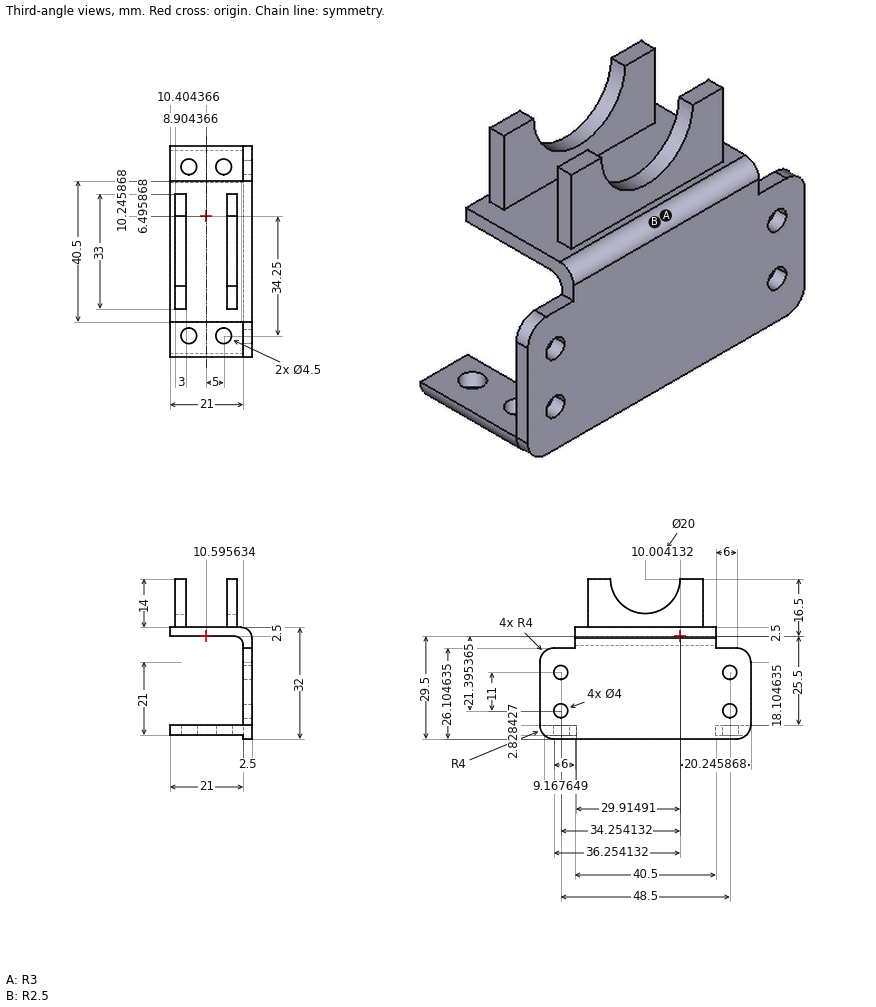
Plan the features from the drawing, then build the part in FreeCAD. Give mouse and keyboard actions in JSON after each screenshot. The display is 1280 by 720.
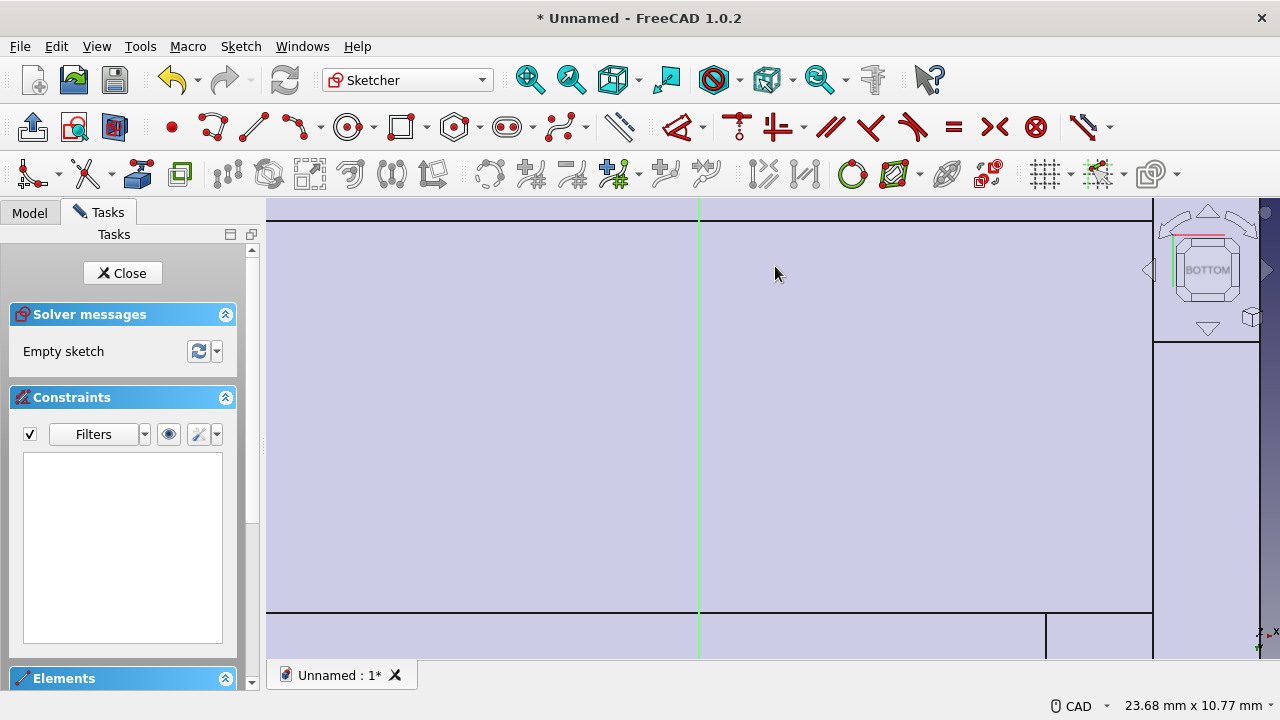
{"action": "left_click", "coordinate": [348, 128]}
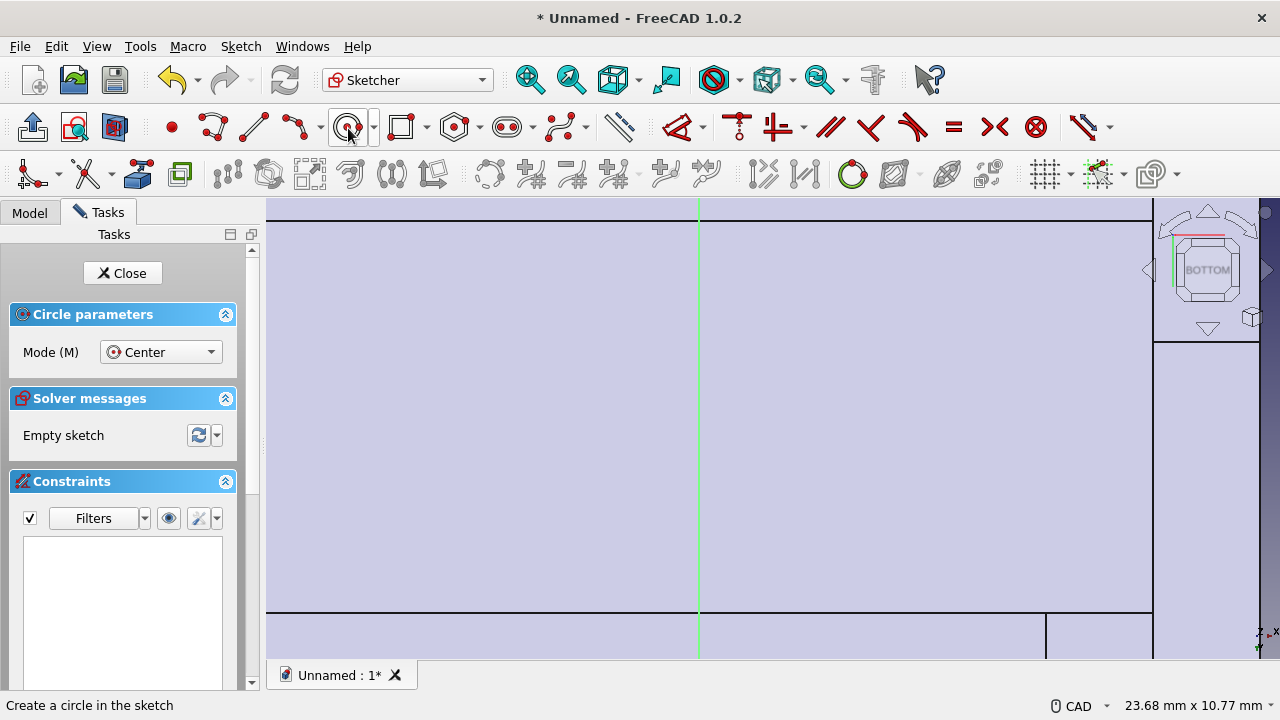
{"action": "left_click", "coordinate": [913, 428]}
{"action": "left_click", "coordinate": [982, 359]}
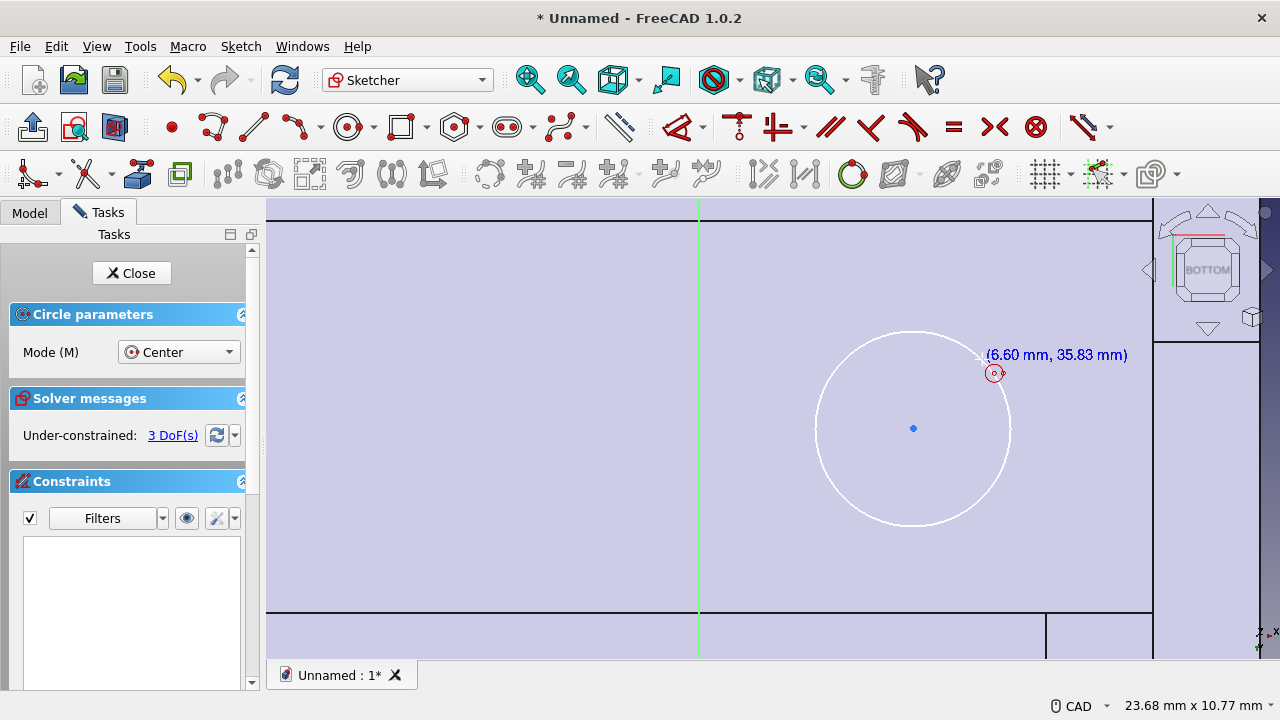
{"action": "left_click", "coordinate": [485, 428]}
{"action": "left_click", "coordinate": [553, 359]}
{"action": "key", "text": "Escape"}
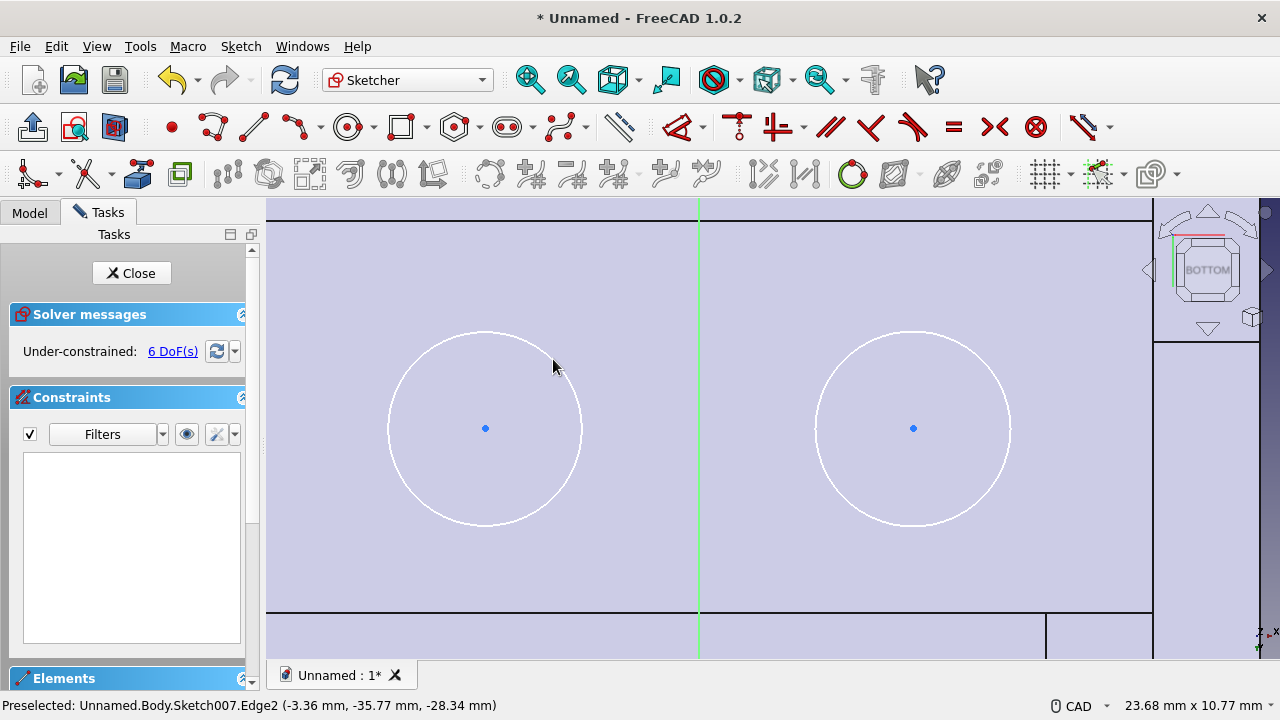
{"action": "left_click", "coordinate": [982, 360]}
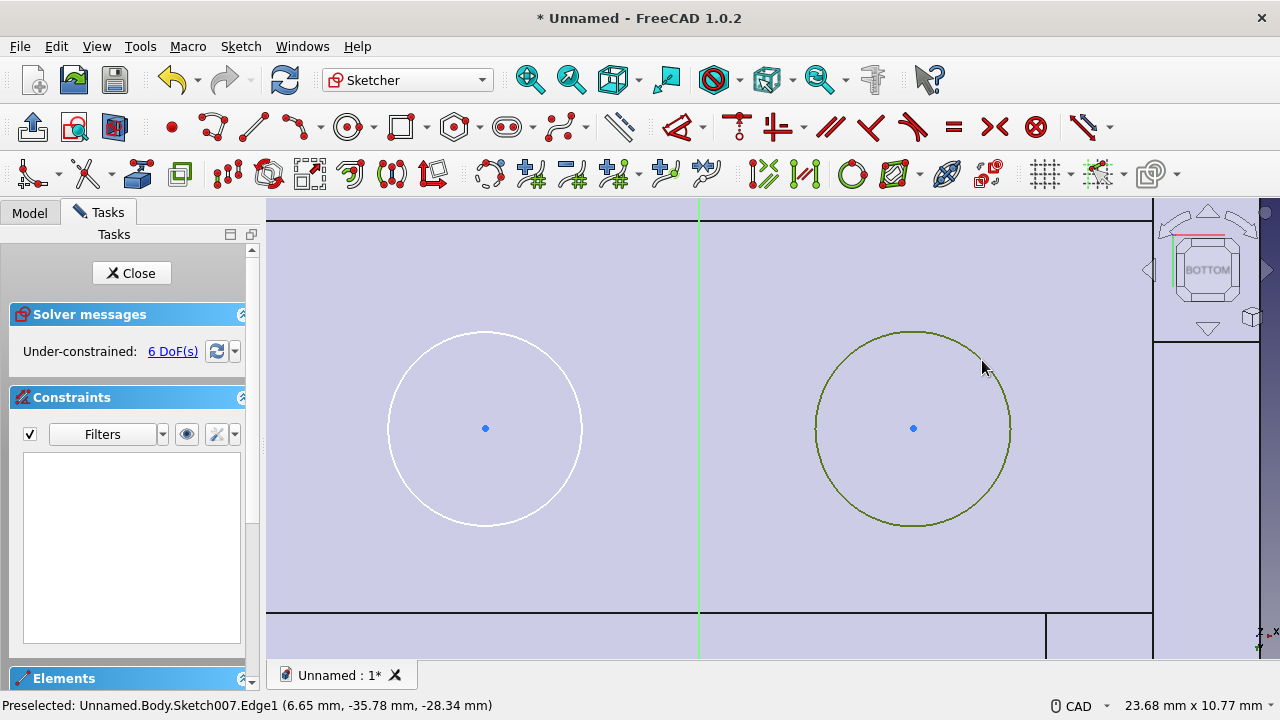
{"action": "left_click", "coordinate": [553, 360]}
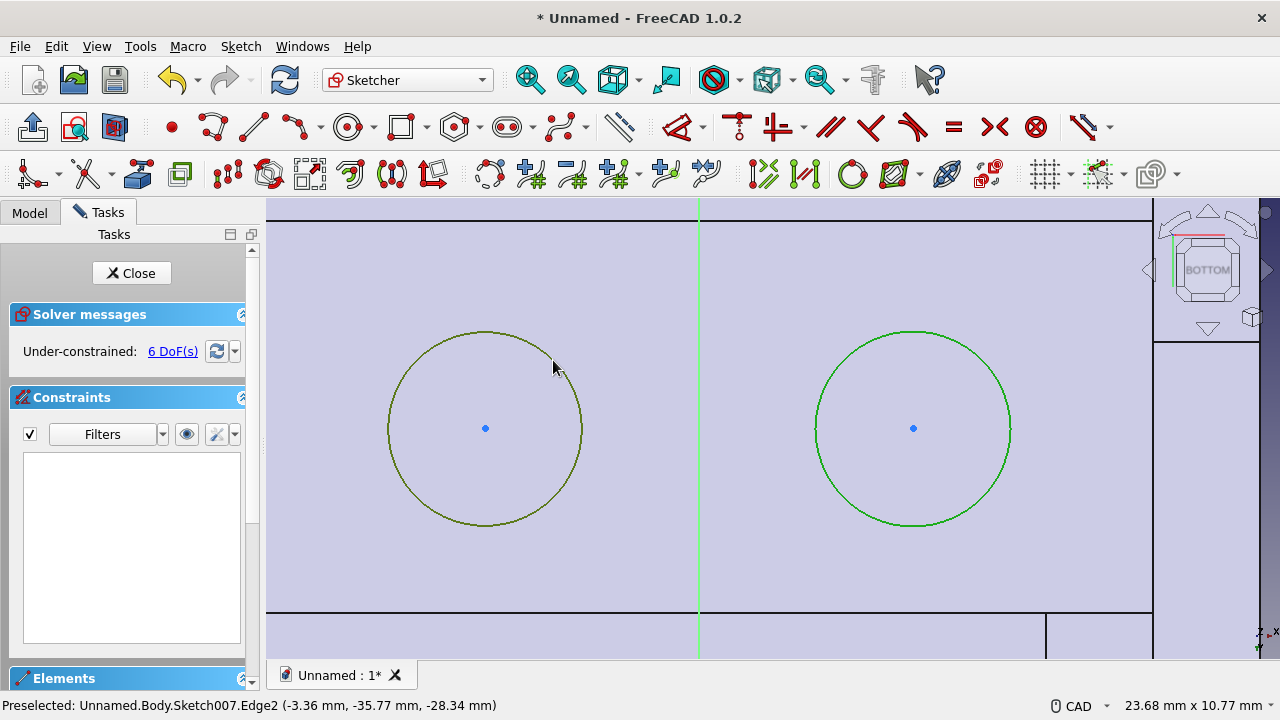
{"action": "left_click", "coordinate": [954, 128]}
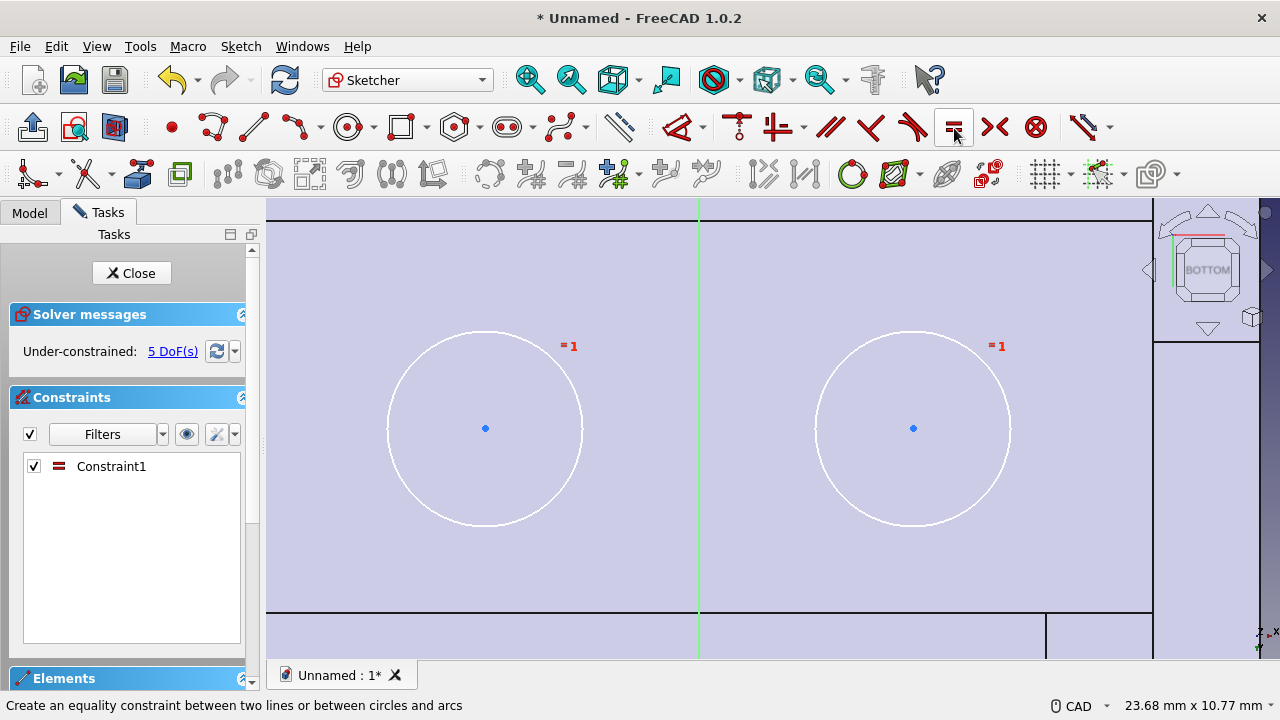
{"action": "left_click", "coordinate": [913, 429]}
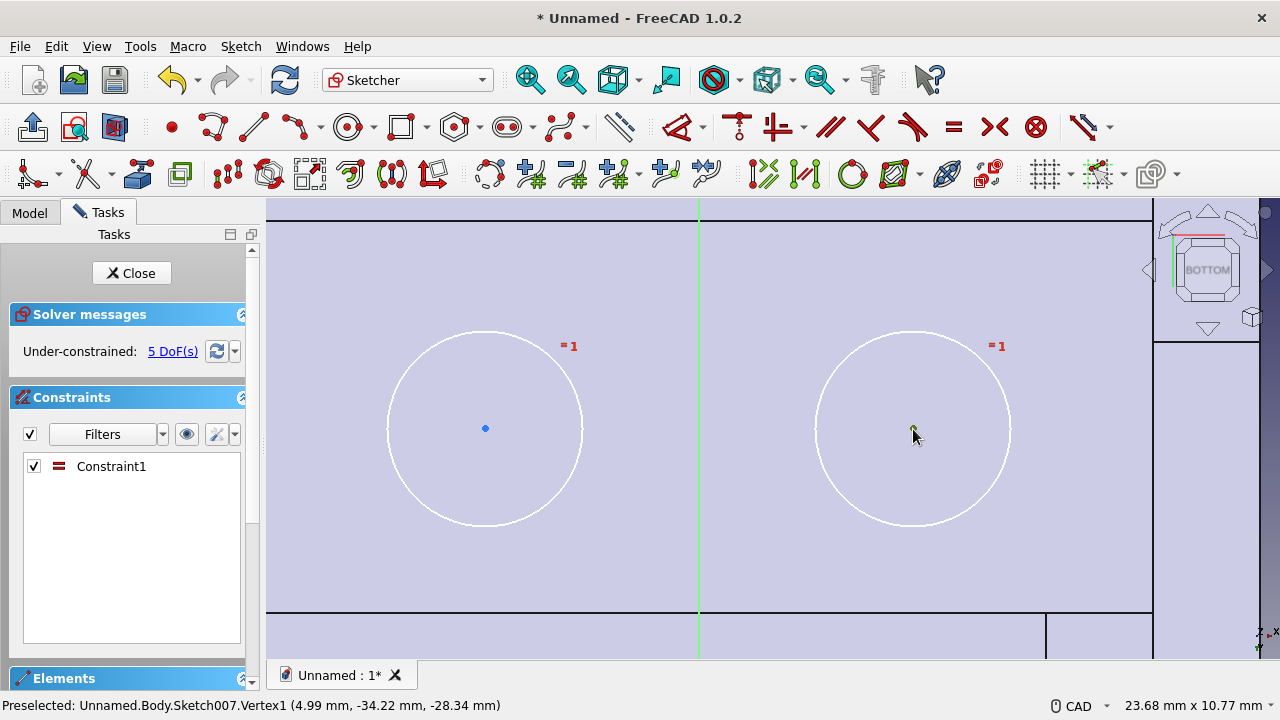
{"action": "left_click", "coordinate": [485, 429]}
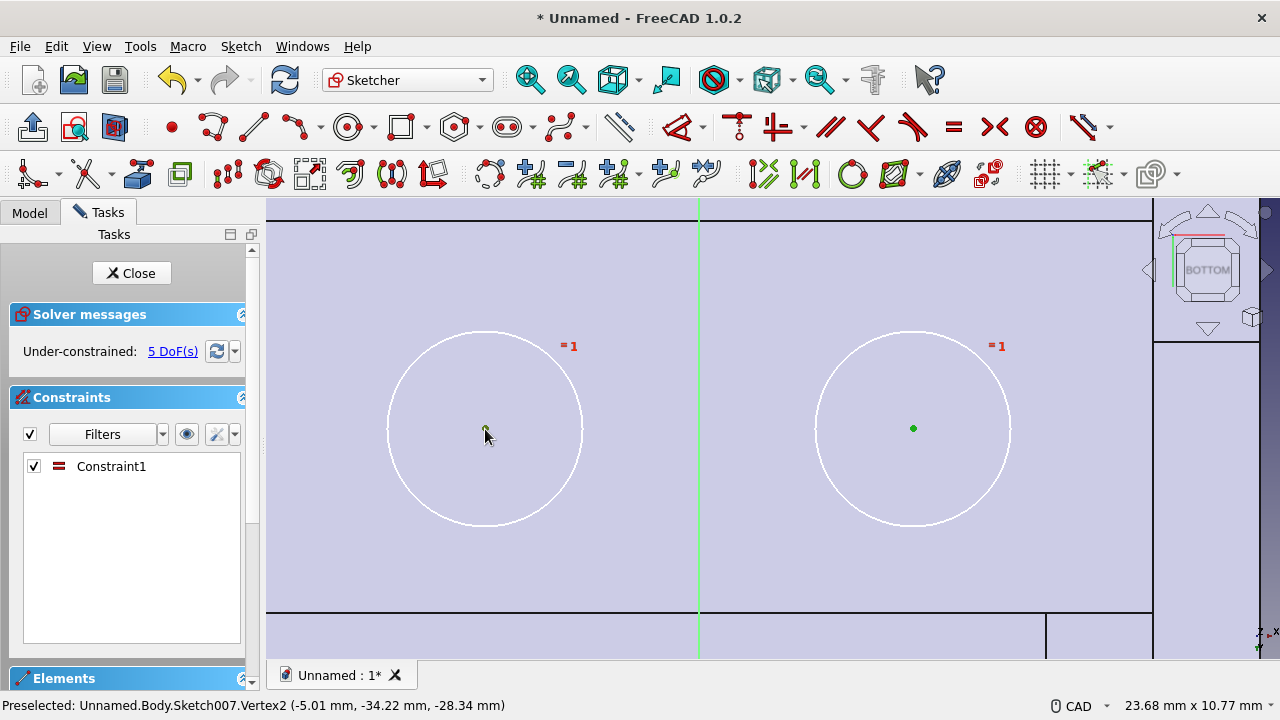
{"action": "left_click", "coordinate": [699, 602]}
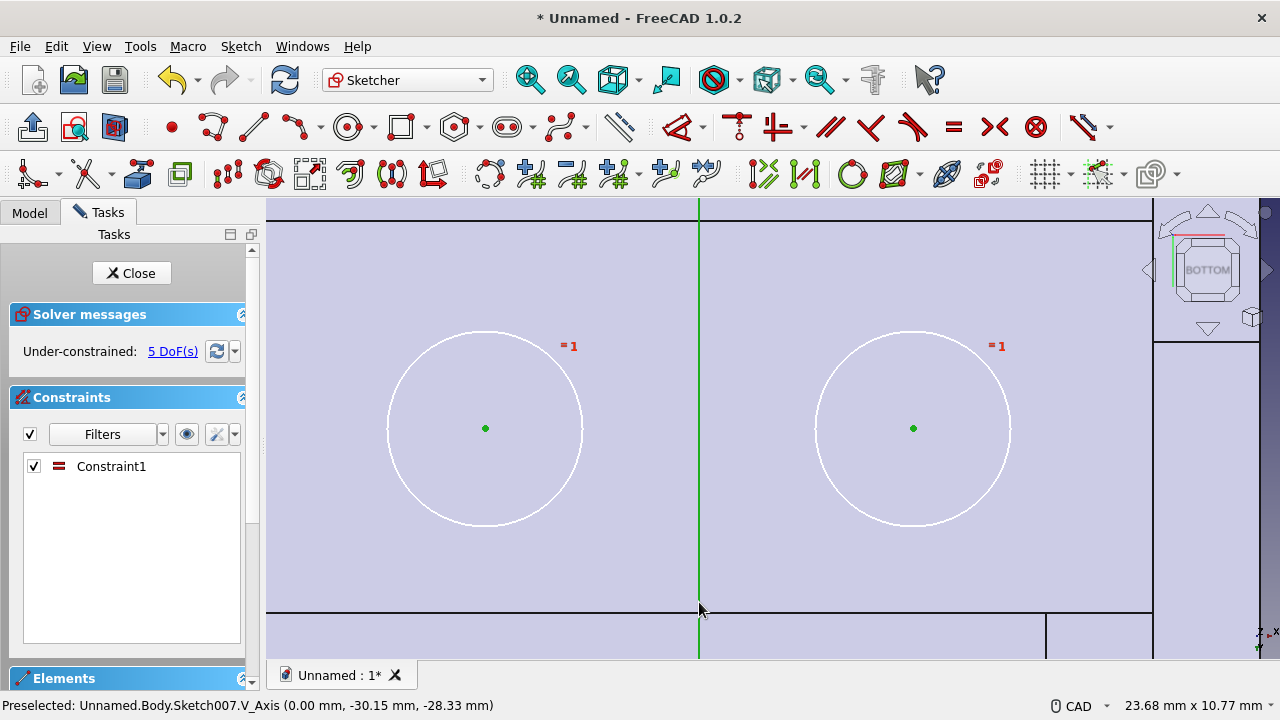
{"action": "left_click", "coordinate": [995, 128]}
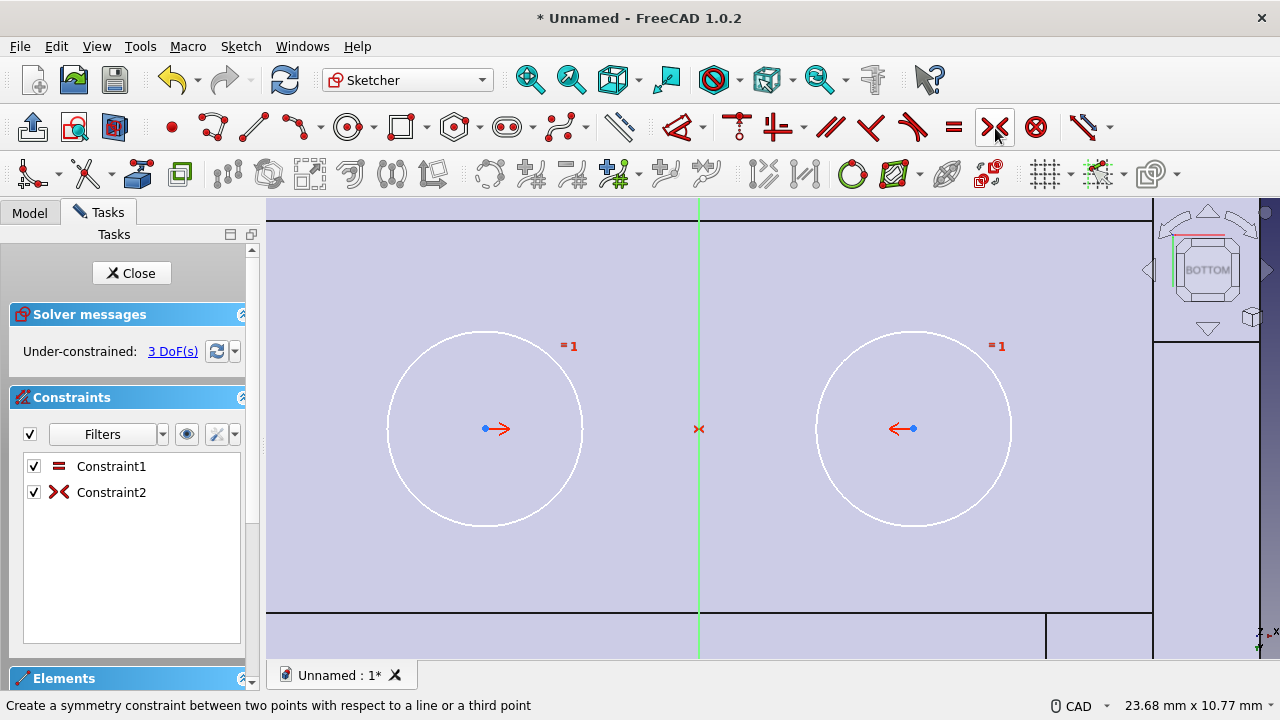
{"action": "left_click", "coordinate": [676, 128]}